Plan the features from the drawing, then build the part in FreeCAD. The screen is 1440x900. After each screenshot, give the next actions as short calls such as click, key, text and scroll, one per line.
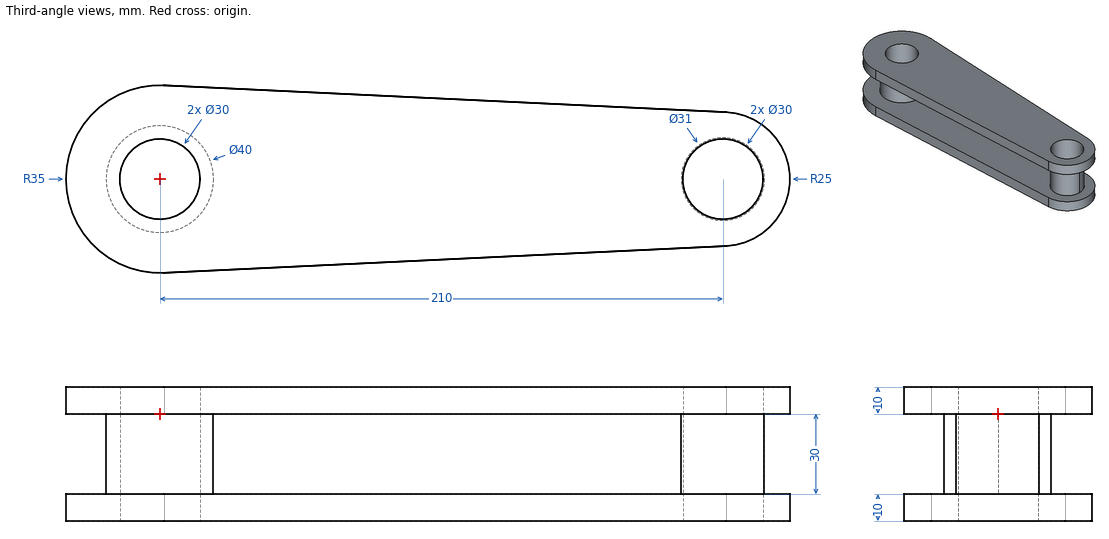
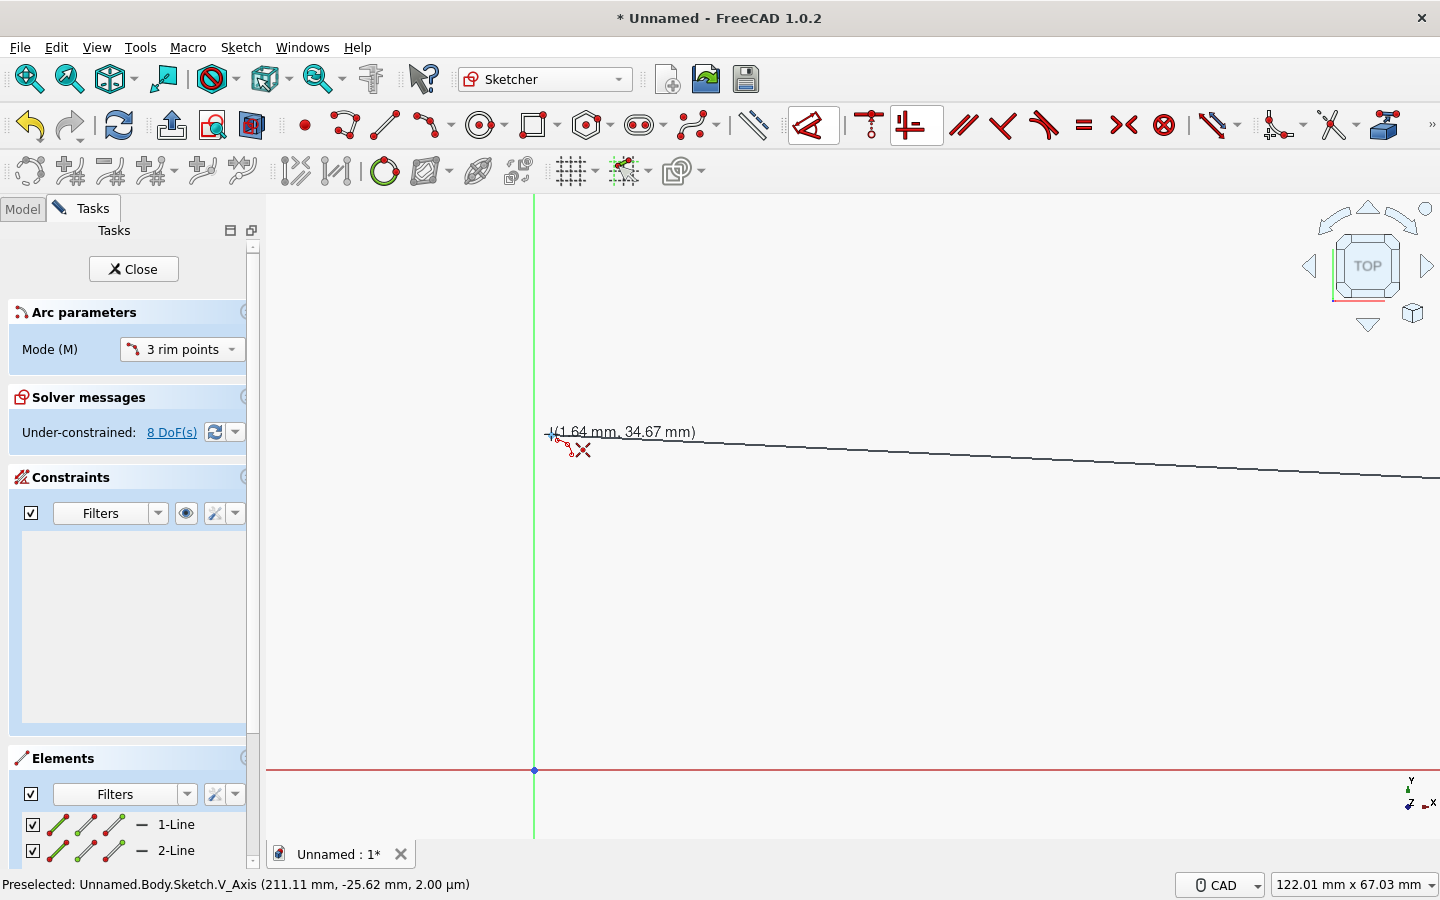
click(551, 435)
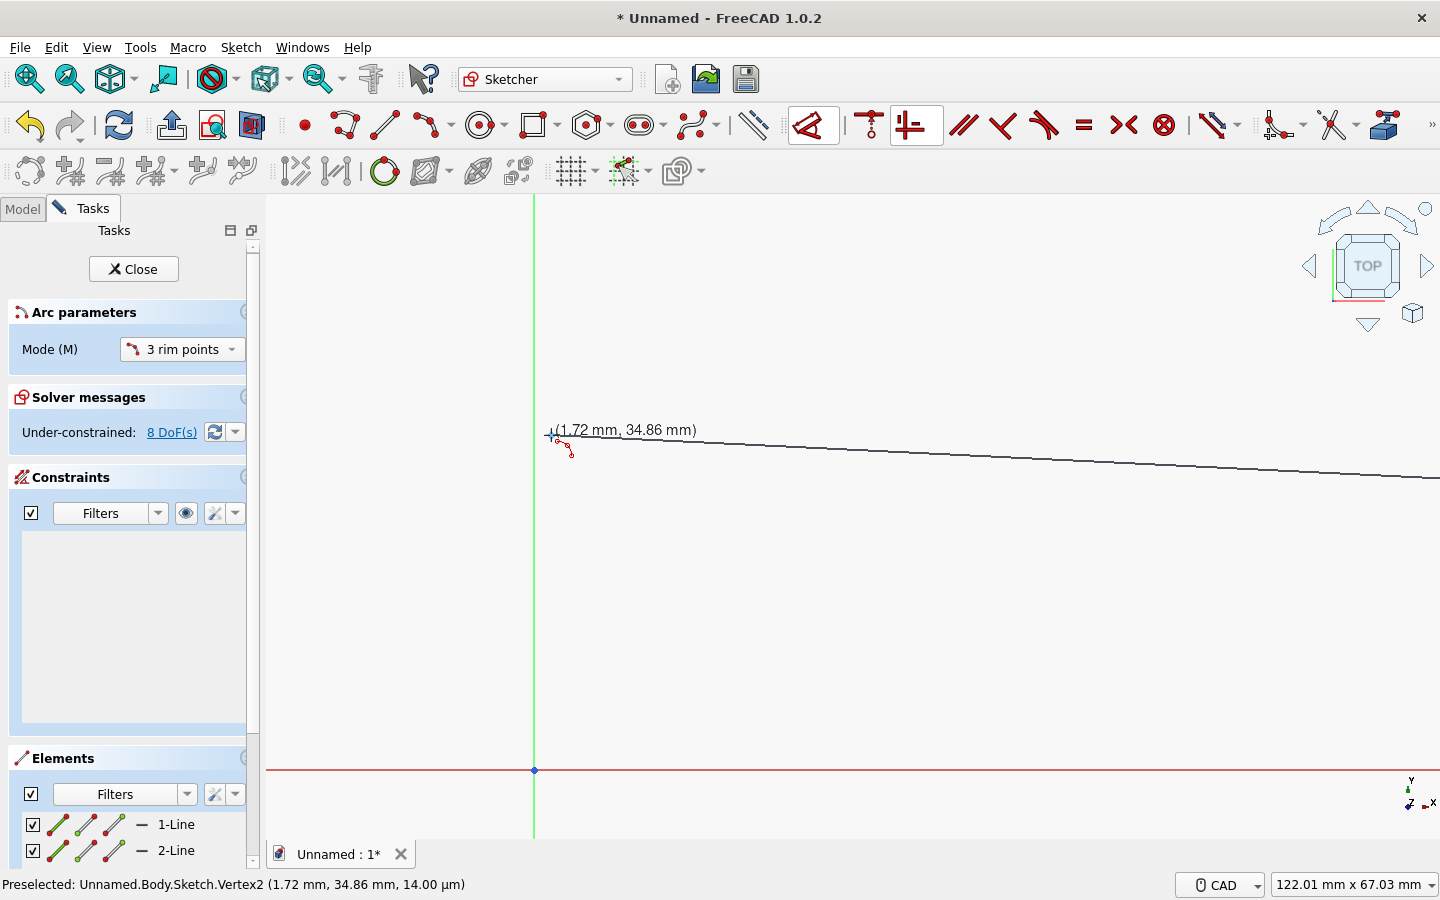
scroll(551, 433, down, 7)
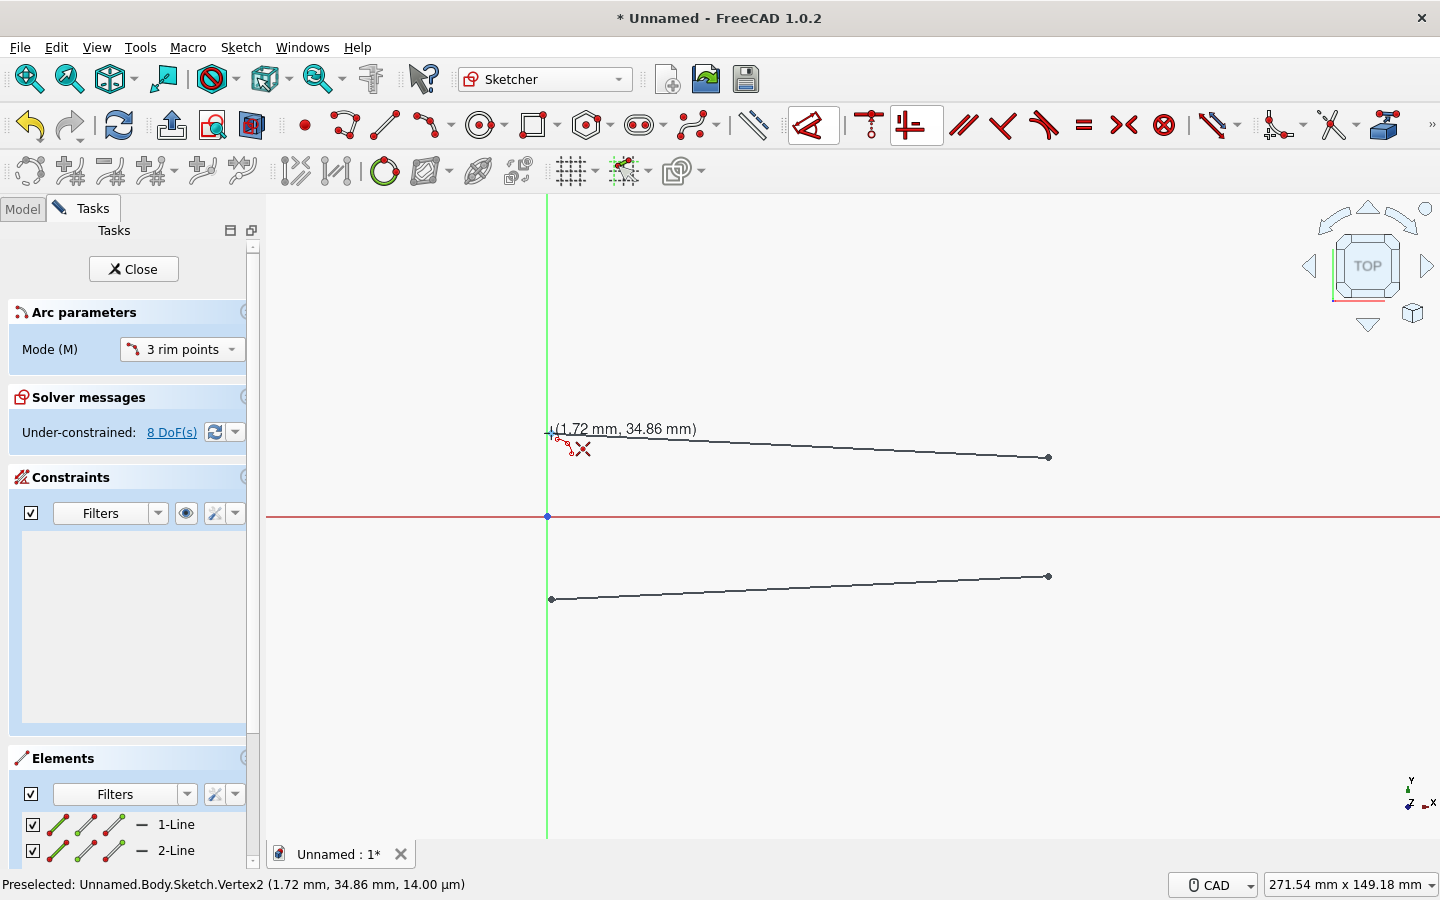
scroll(551, 599, up, 7)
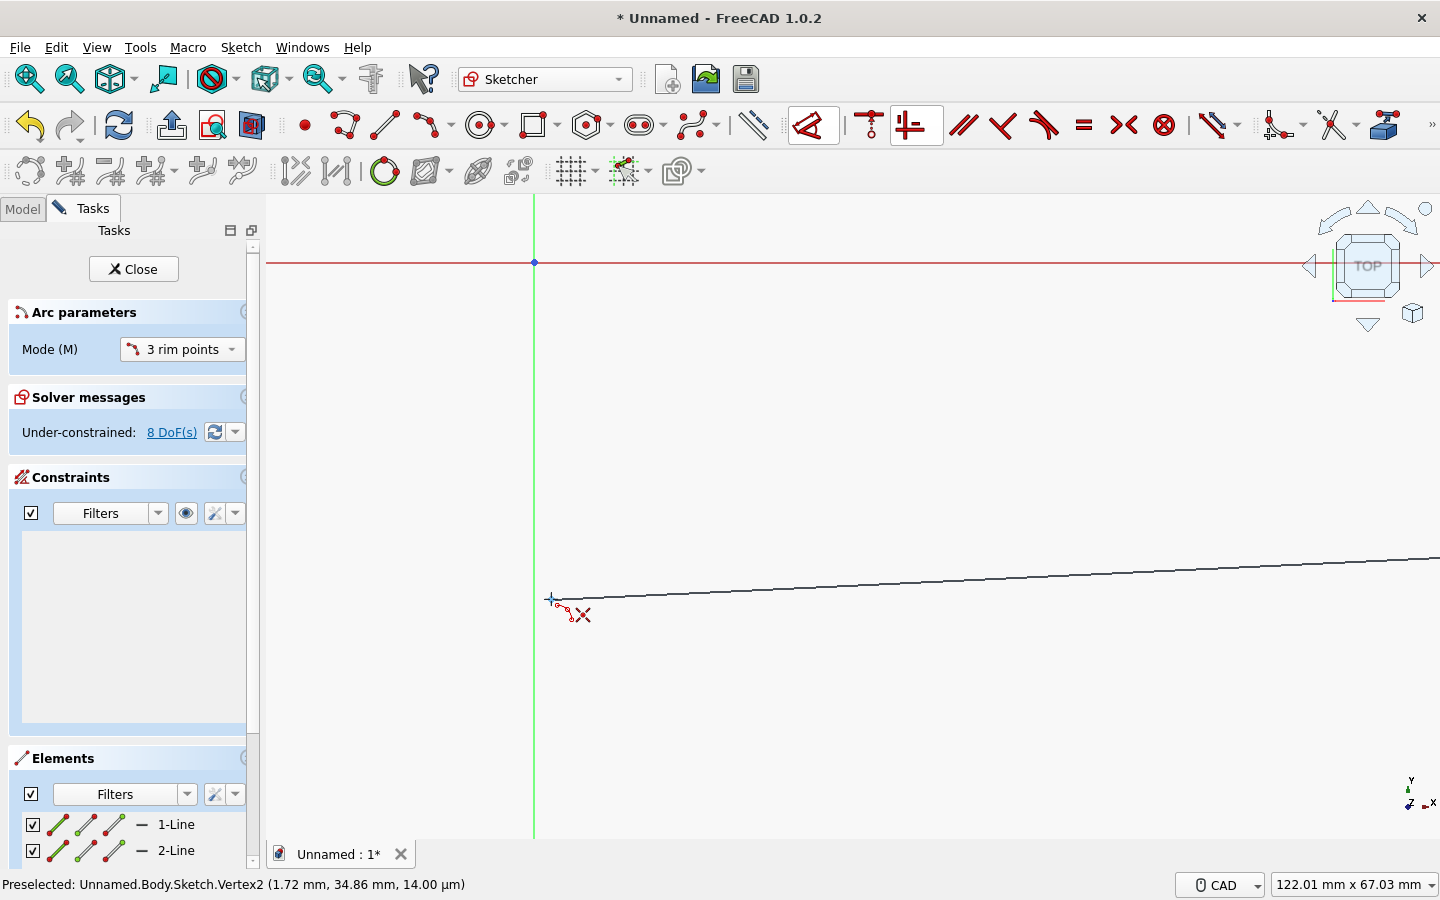
click(551, 600)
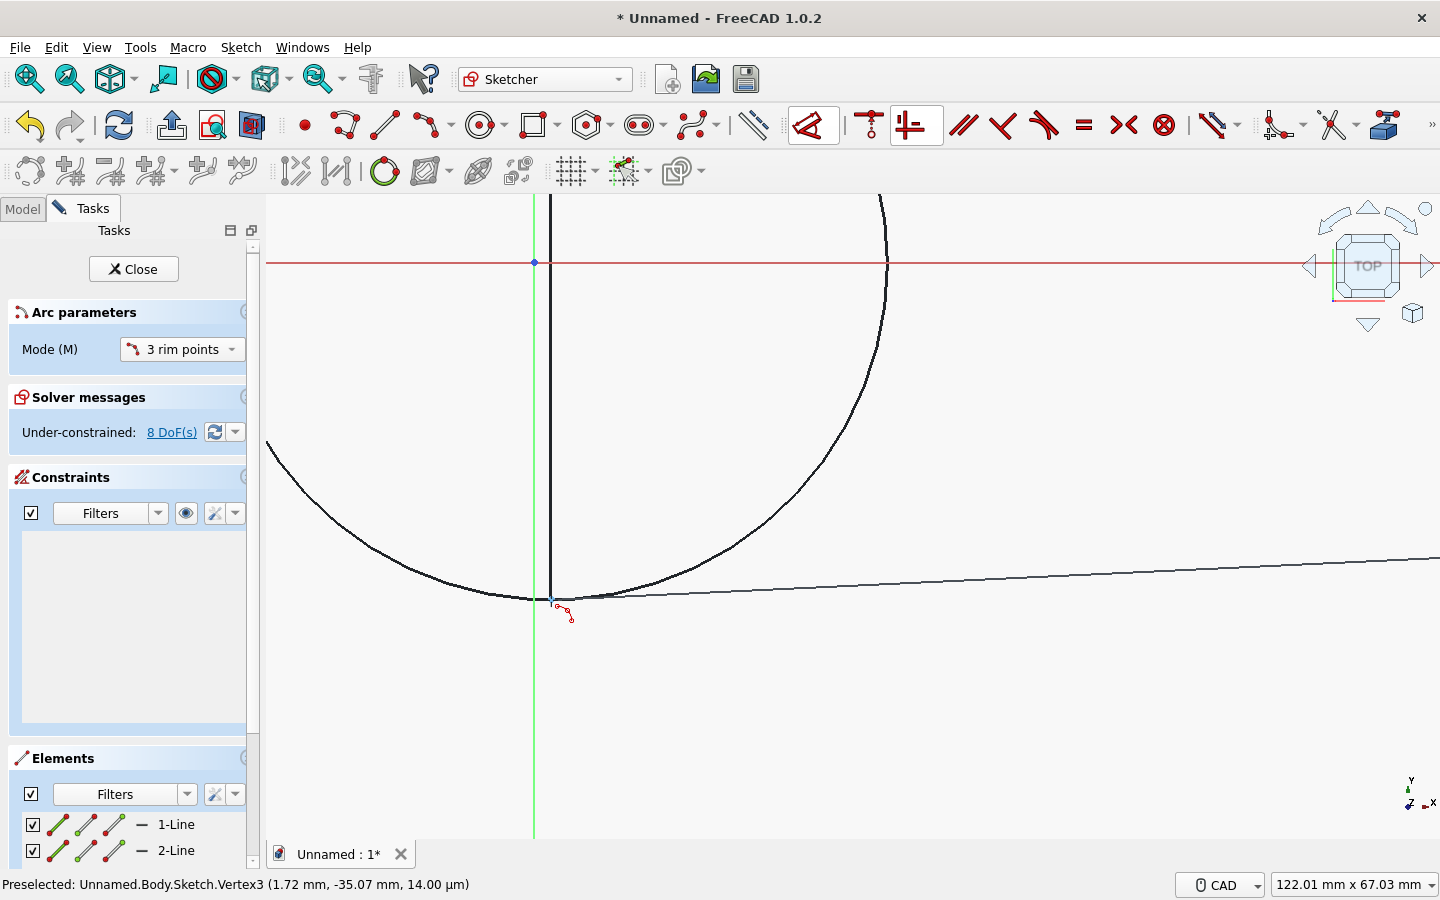
scroll(551, 600, down, 7)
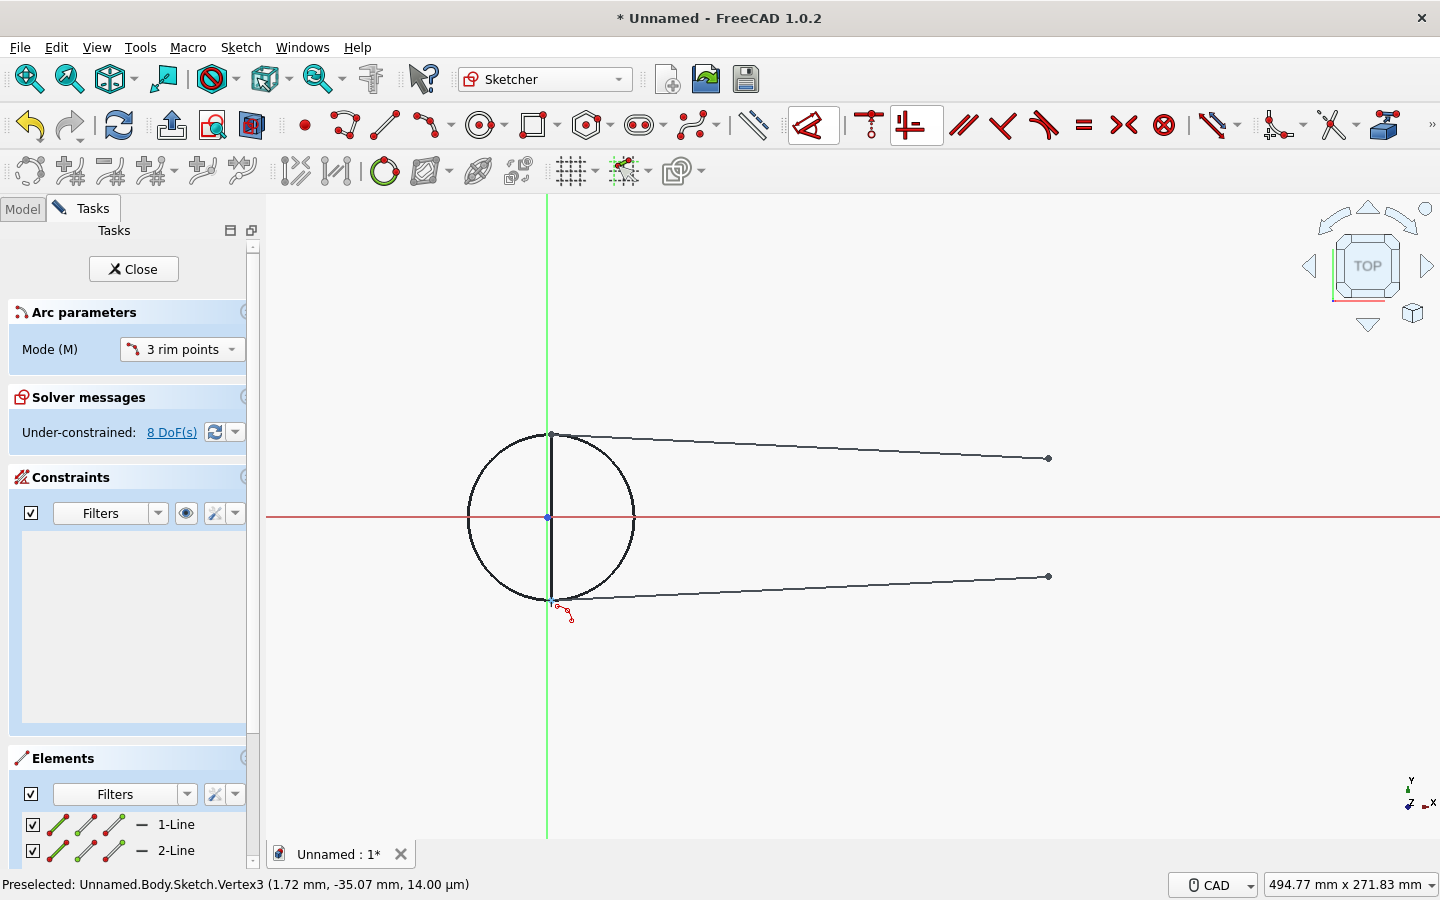
click(468, 491)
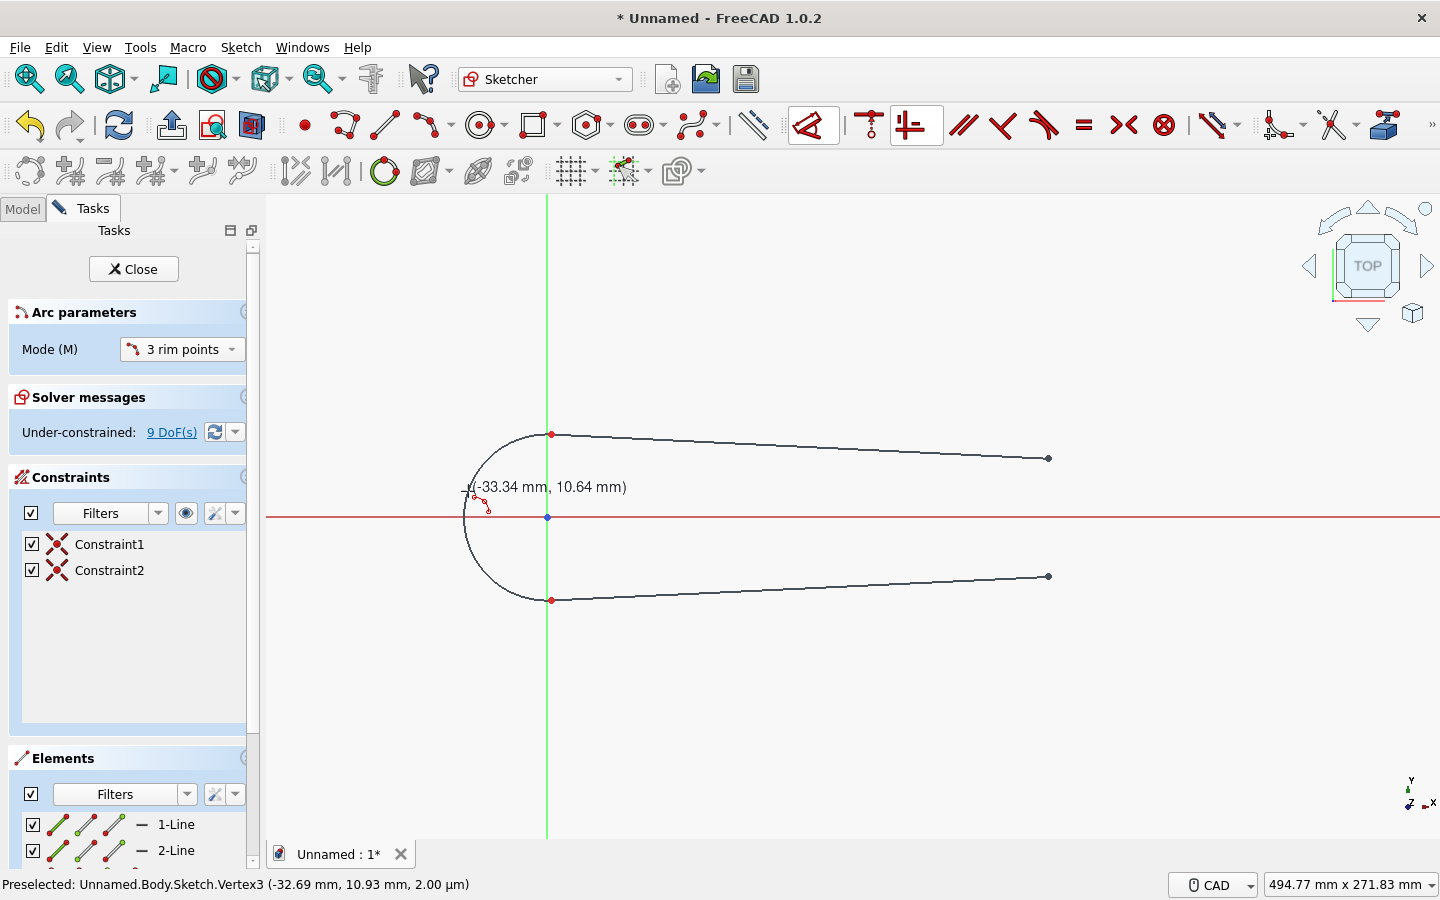
click(1048, 577)
click(1048, 459)
click(1102, 535)
key(Escape)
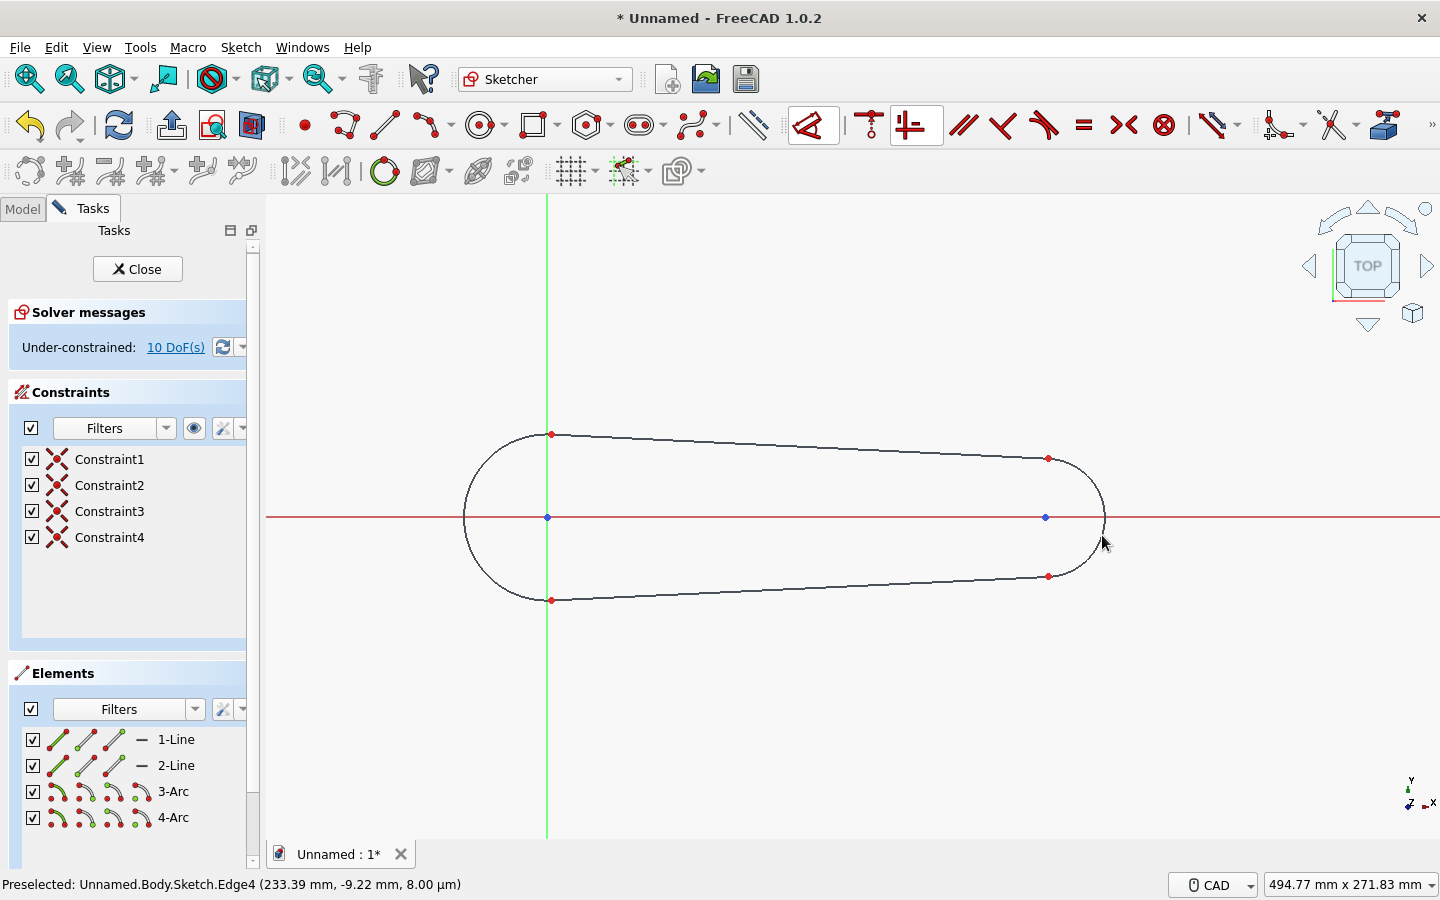
click(899, 451)